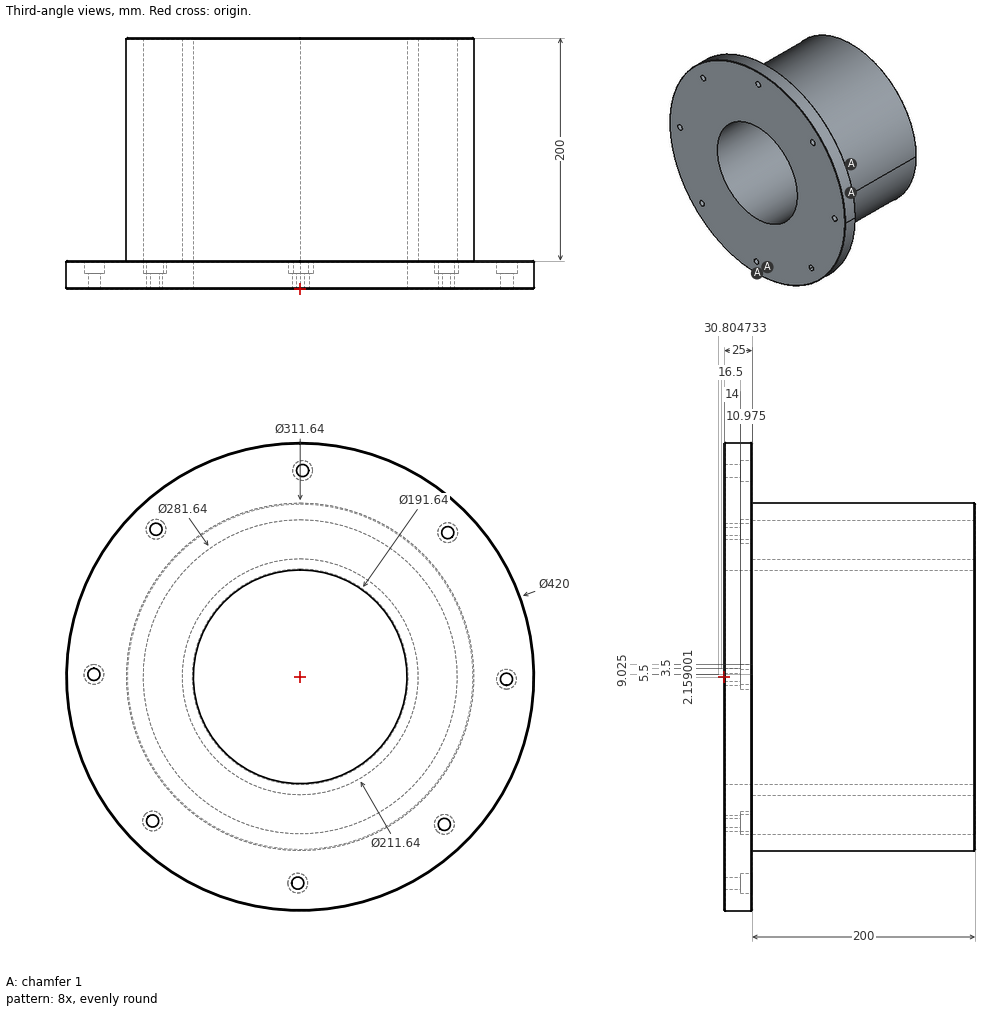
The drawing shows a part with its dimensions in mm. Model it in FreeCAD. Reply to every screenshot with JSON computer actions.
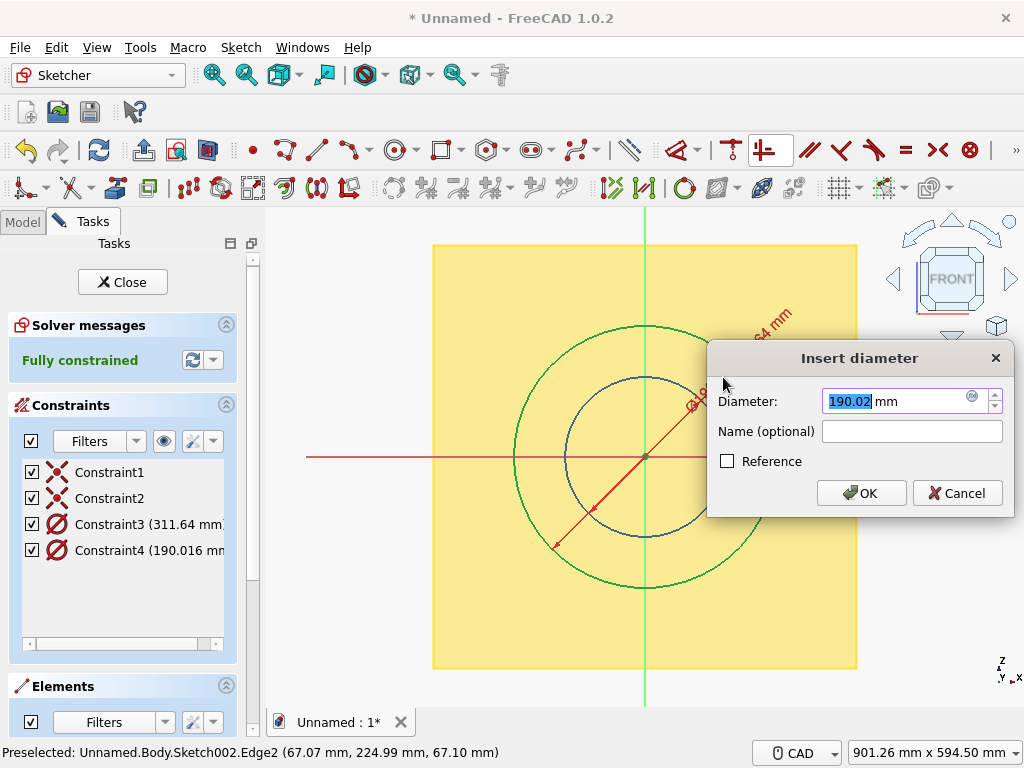
{"action": "type", "text": "191.64"}
{"action": "key", "text": "Return"}
{"action": "key", "text": "Escape"}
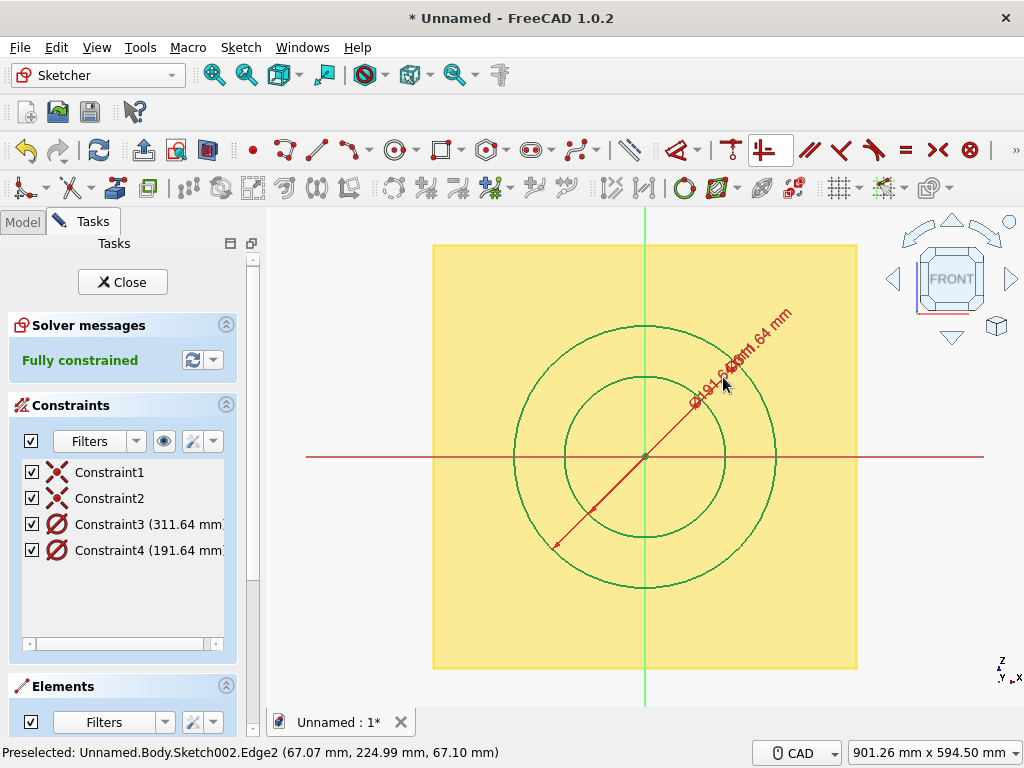
{"action": "left_click", "coordinate": [123, 282]}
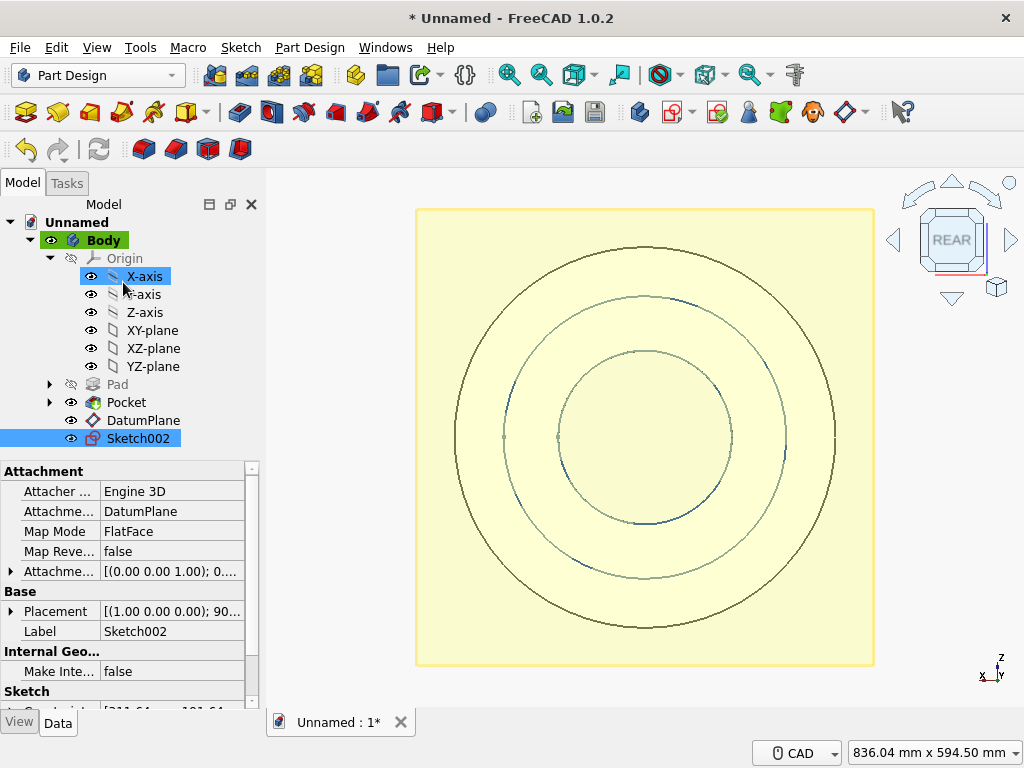
{"action": "left_click", "coordinate": [26, 112]}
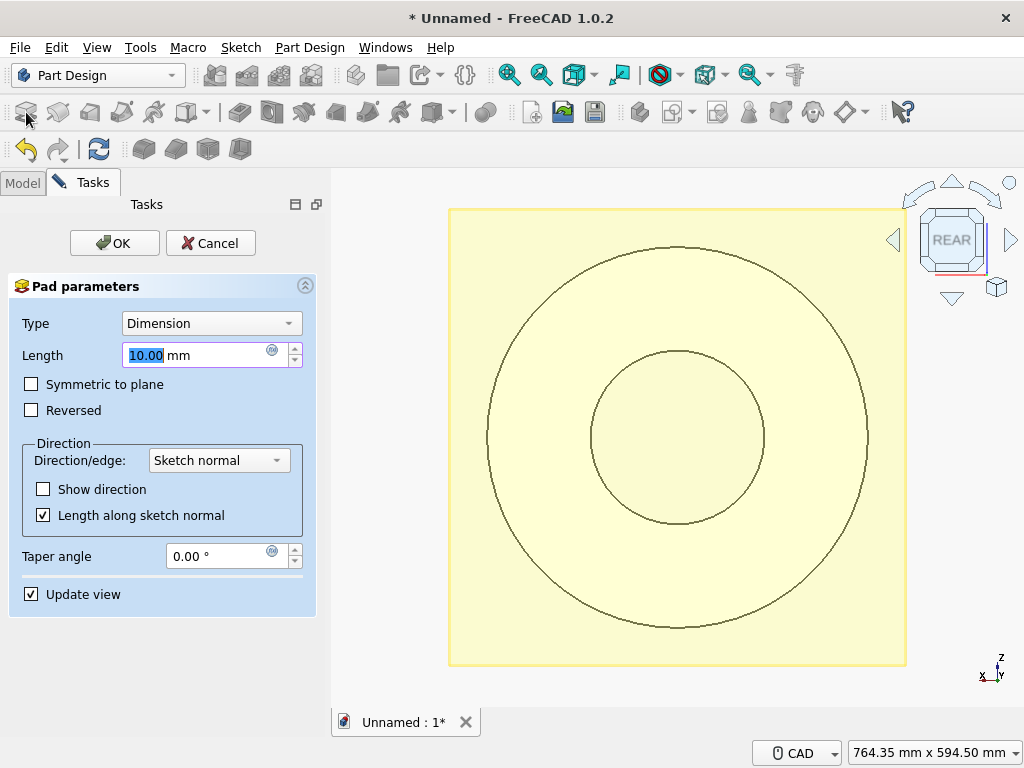
{"action": "type", "text": "200"}
{"action": "key", "text": "Tab"}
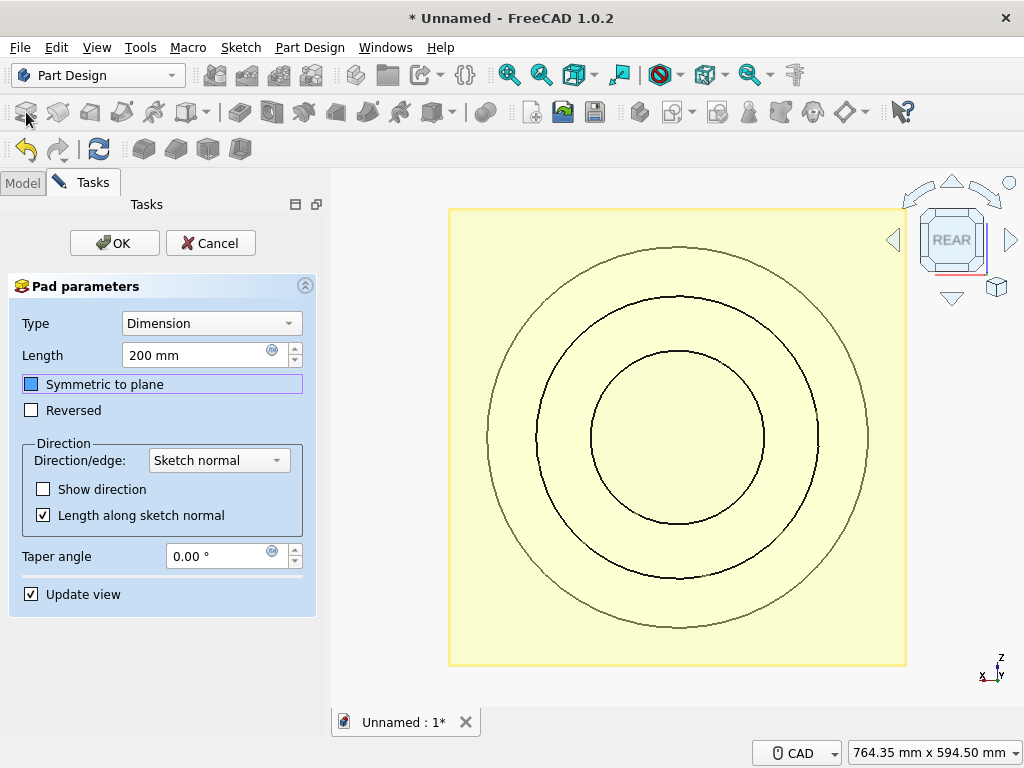
{"action": "left_click", "coordinate": [115, 243]}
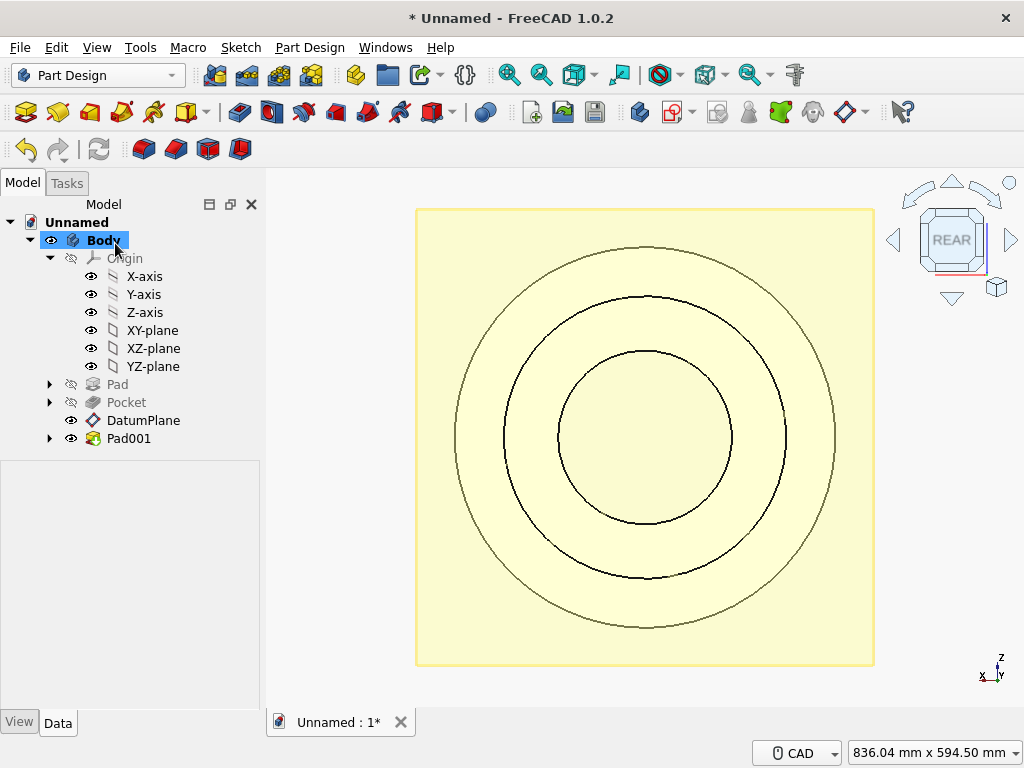
{"action": "left_click", "coordinate": [116, 420]}
{"action": "key", "text": "space"}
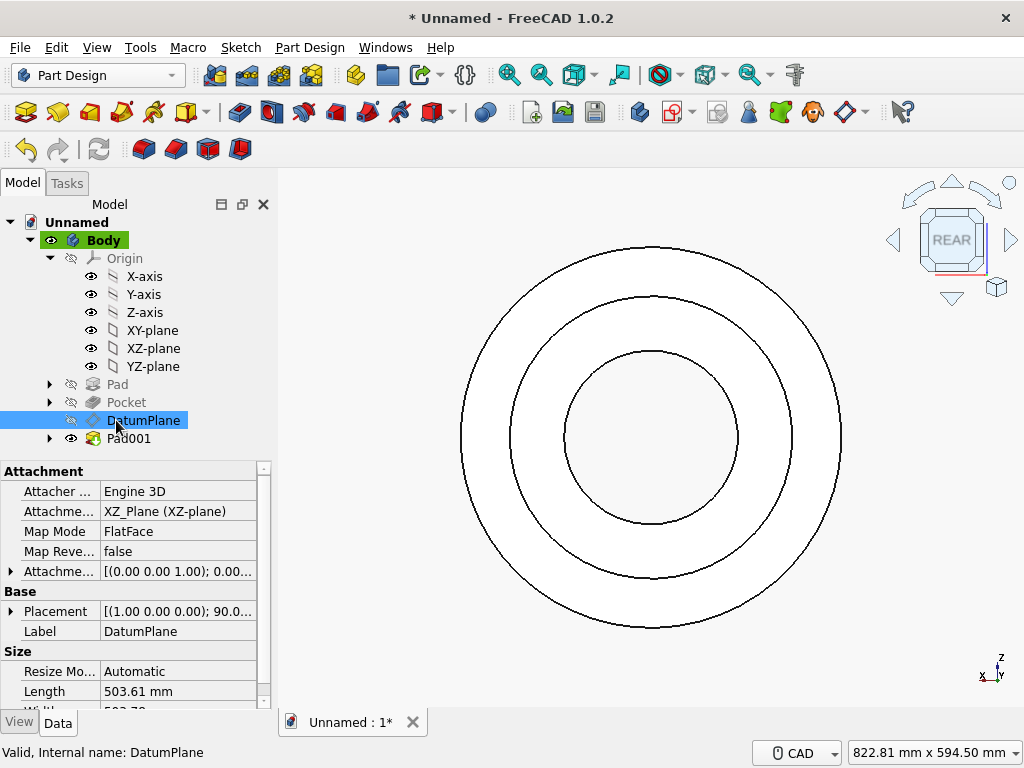
{"action": "left_click", "coordinate": [792, 437]}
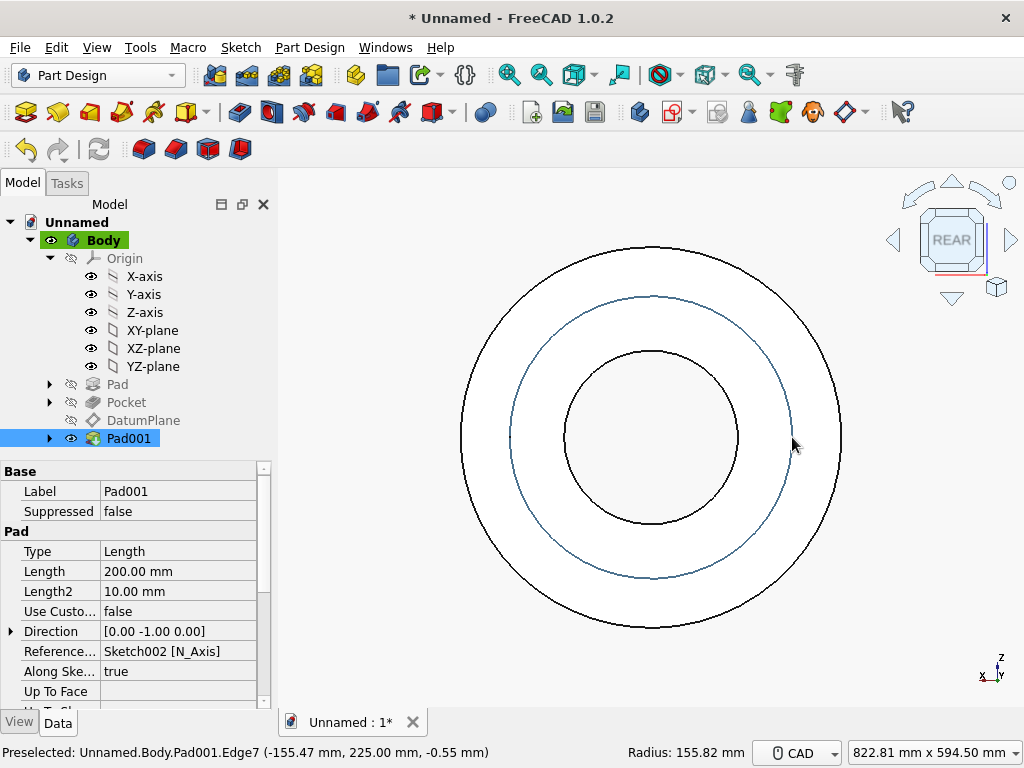
{"action": "left_click", "coordinate": [721, 385], "text": "ctrl"}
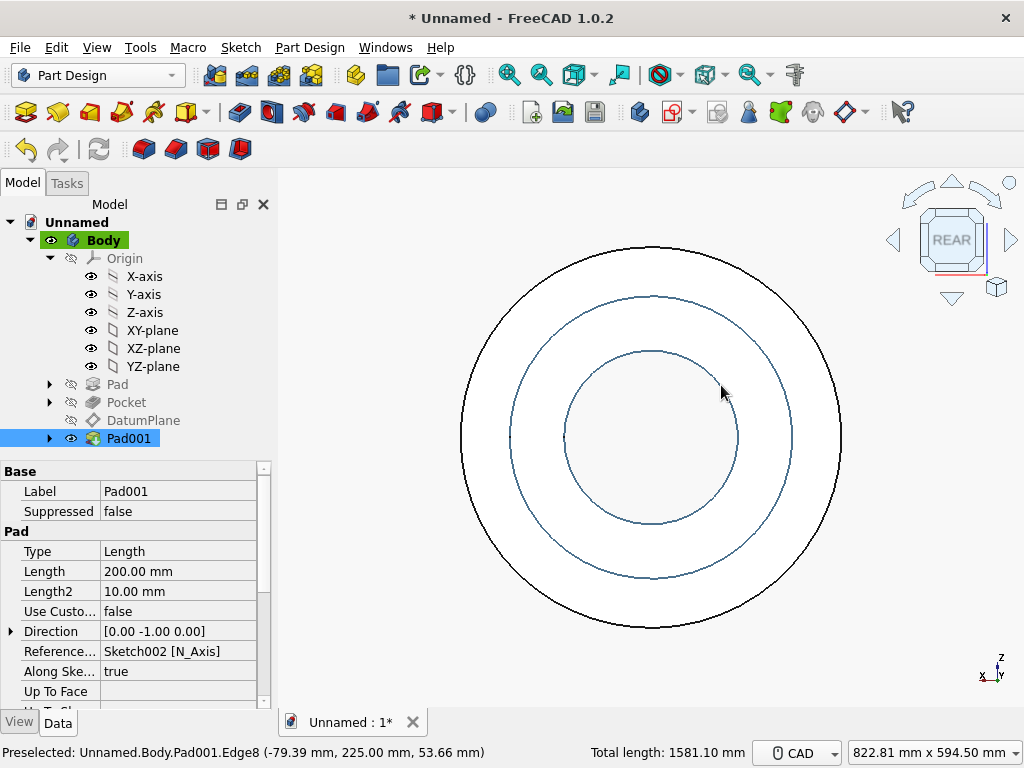
{"action": "left_click", "coordinate": [841, 437], "text": "ctrl"}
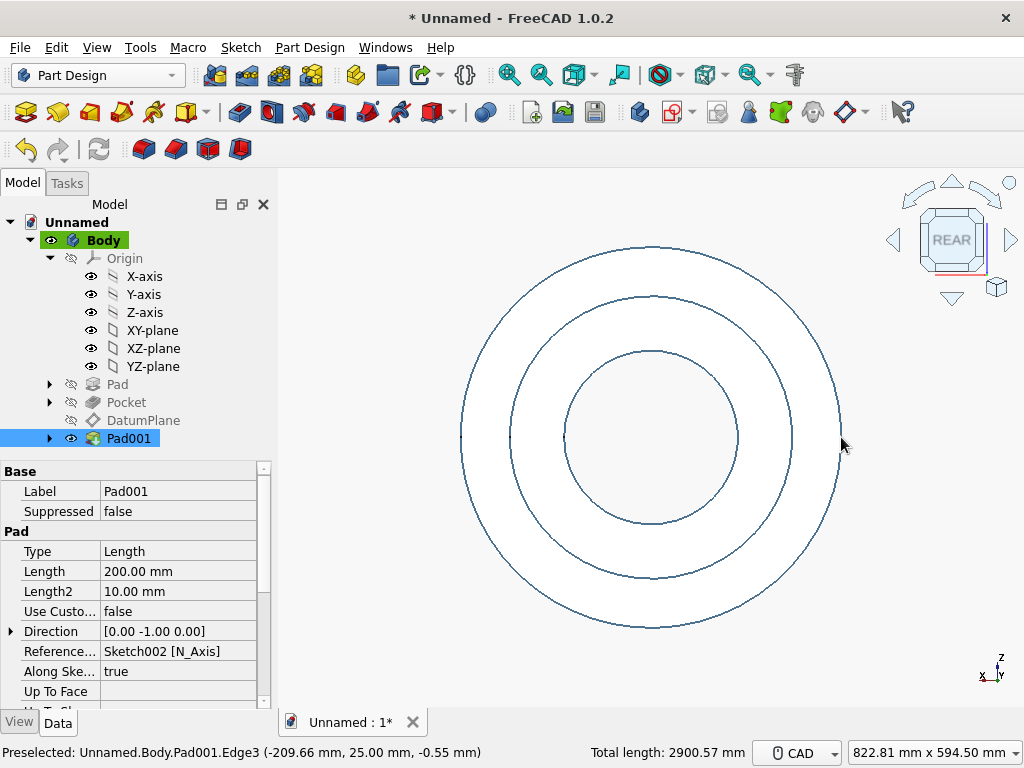
{"action": "key", "text": "0"}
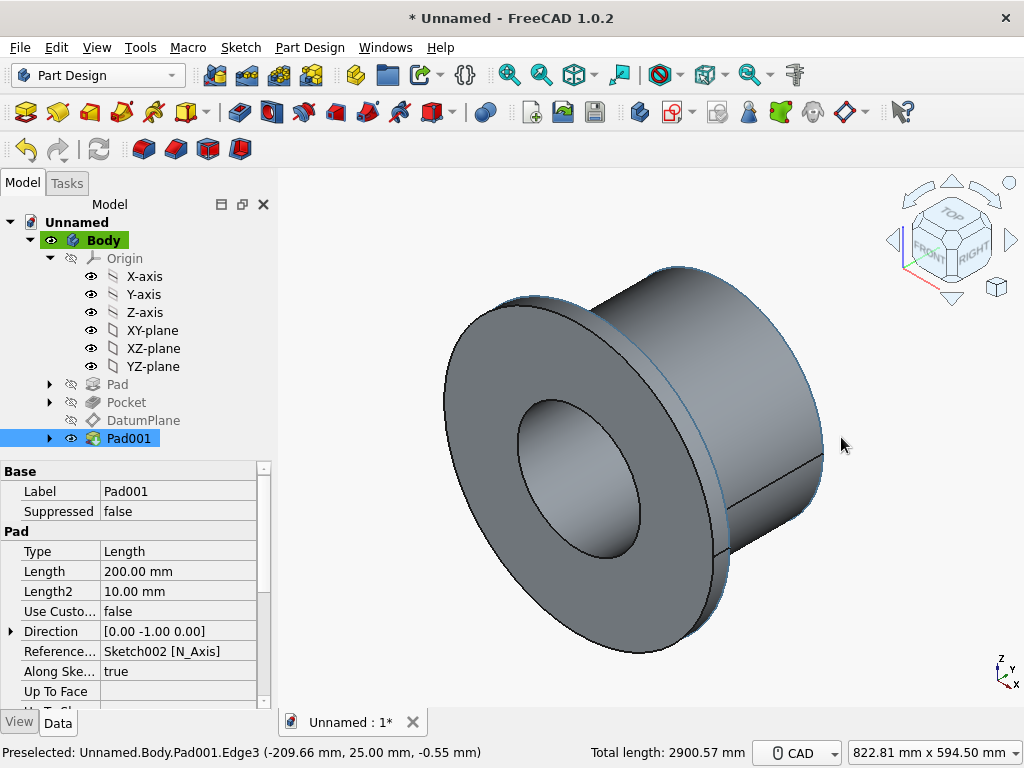
{"action": "left_click", "coordinate": [510, 76]}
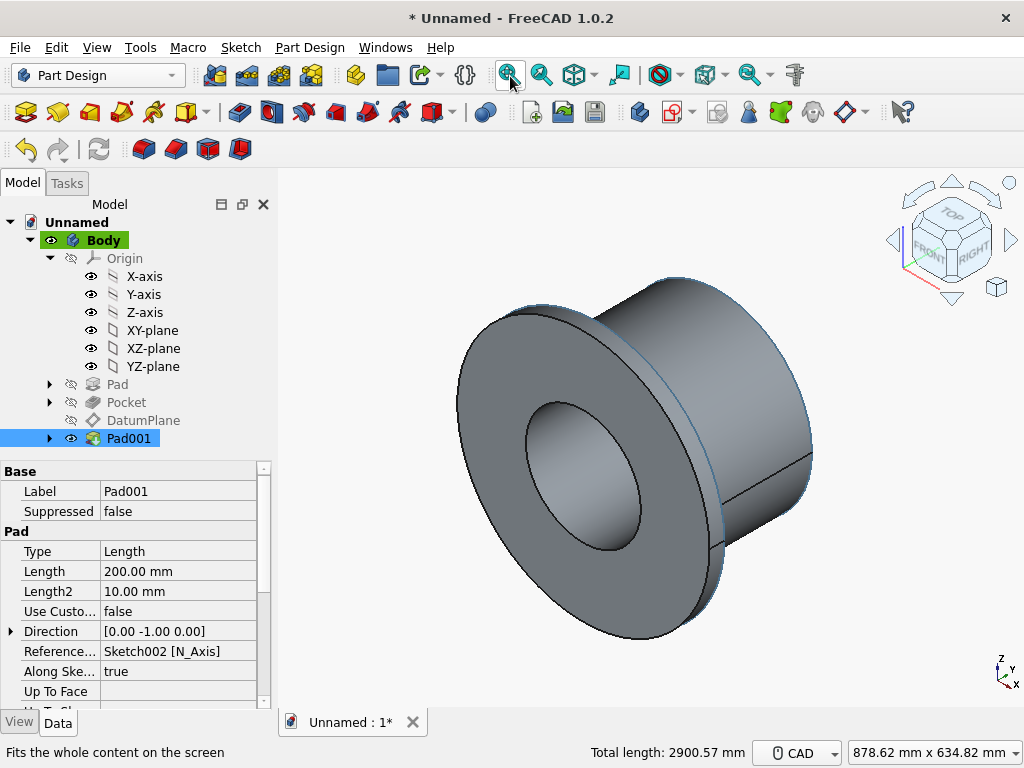
{"action": "left_click", "coordinate": [544, 314], "text": "ctrl"}